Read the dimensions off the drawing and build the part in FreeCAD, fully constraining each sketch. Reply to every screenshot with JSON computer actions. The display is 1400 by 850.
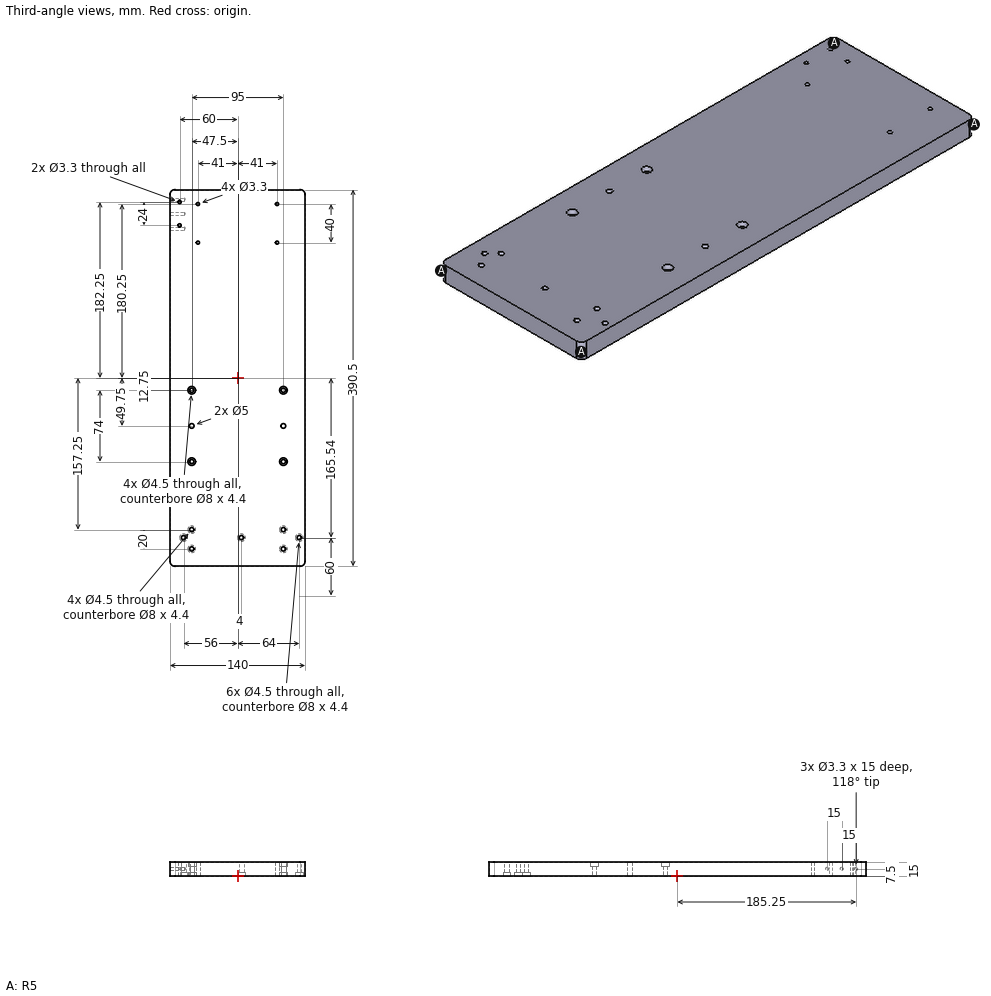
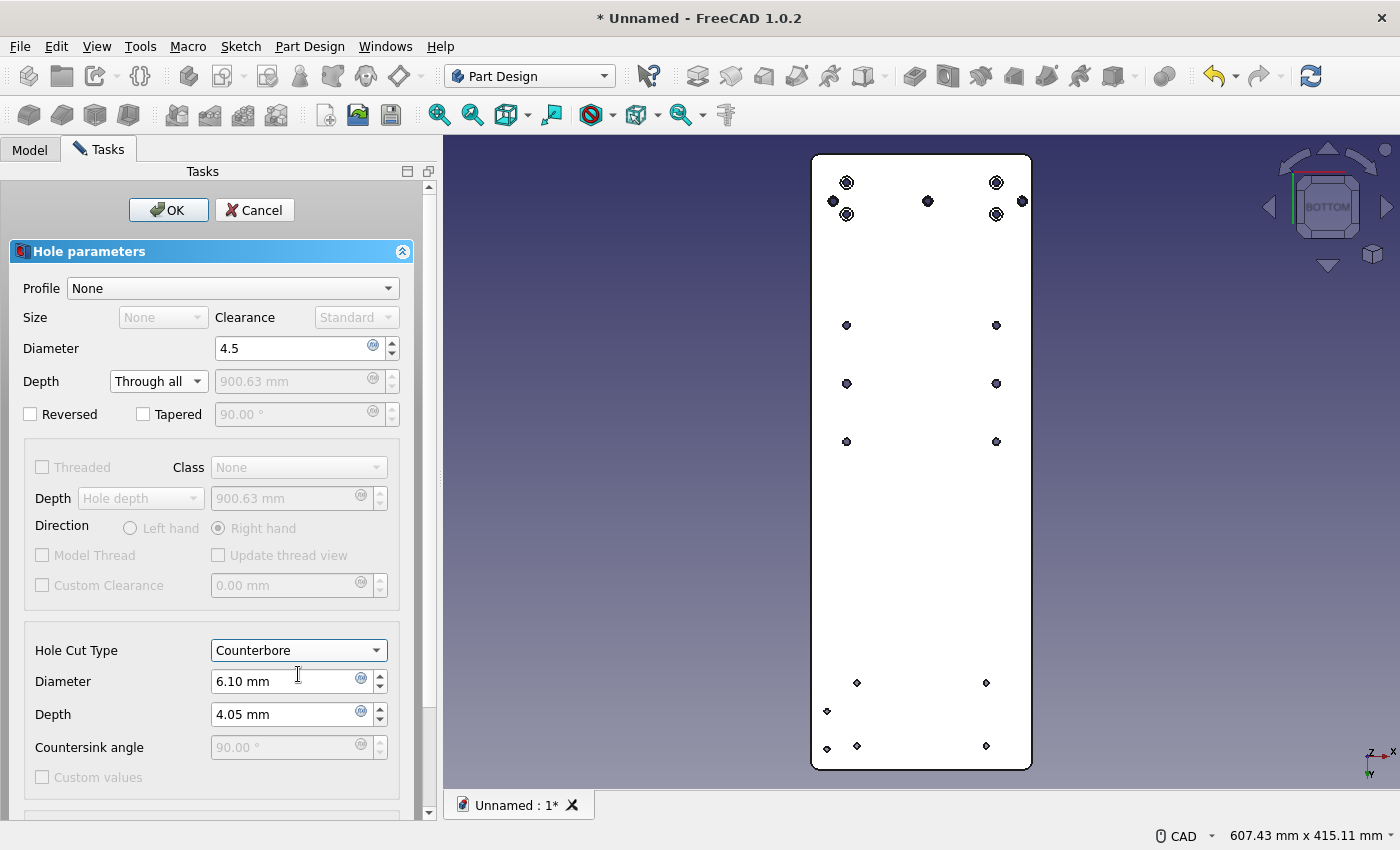
{"action": "triple_click", "coordinate": [292, 682]}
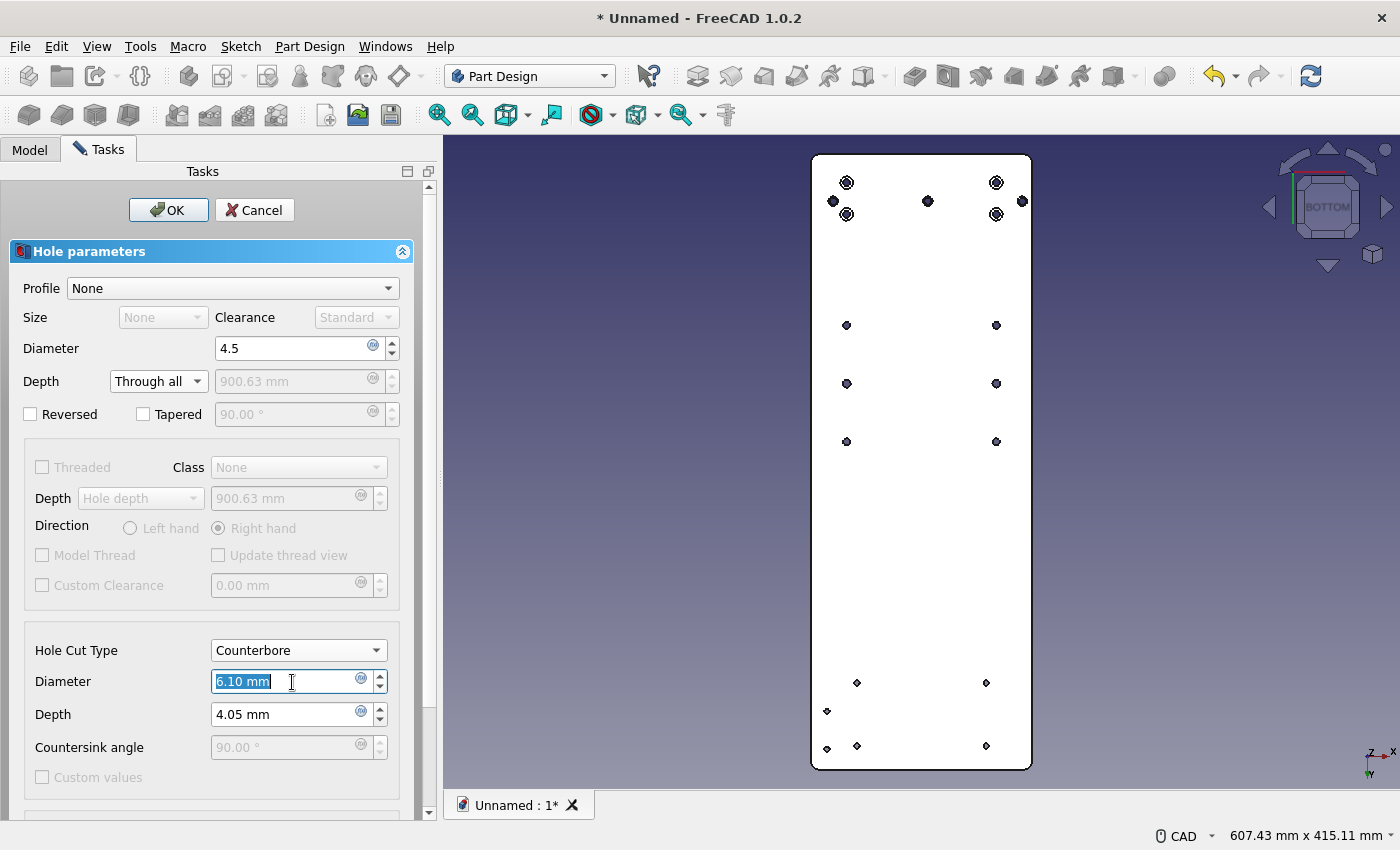
{"action": "type", "text": "8"}
{"action": "key", "text": "Tab"}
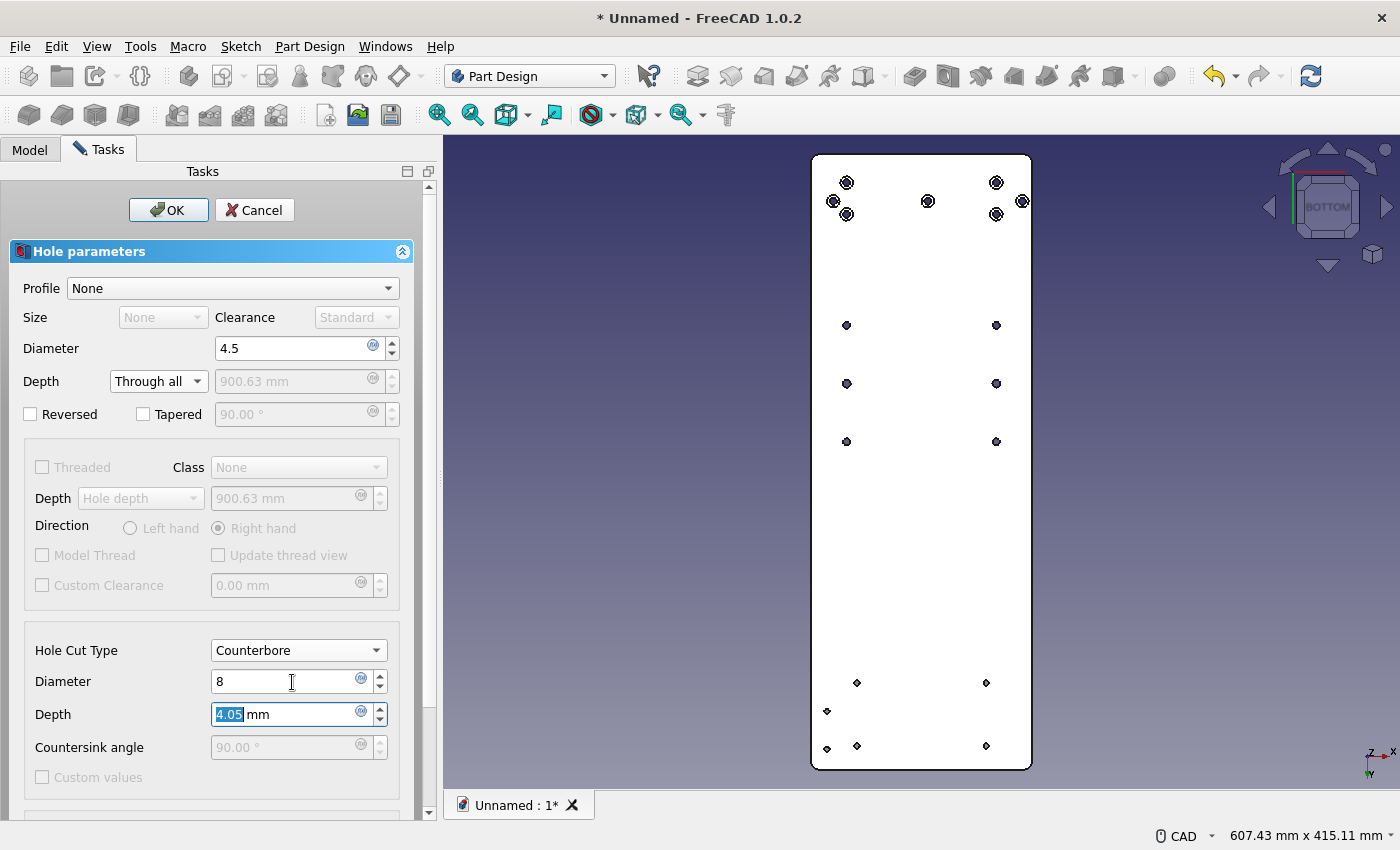
{"action": "type", "text": "4.4"}
{"action": "key", "text": "Tab"}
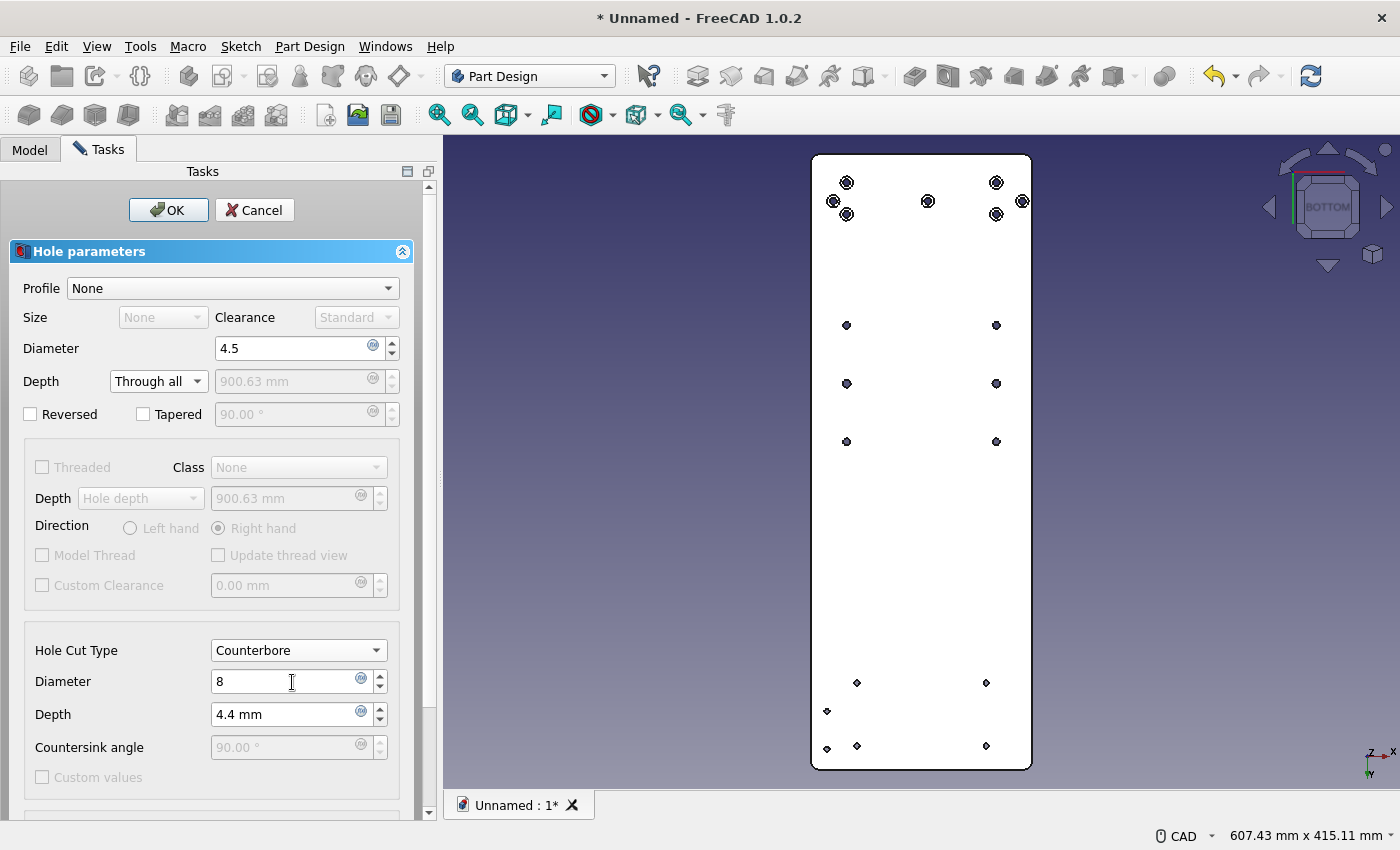
{"action": "left_click", "coordinate": [169, 210]}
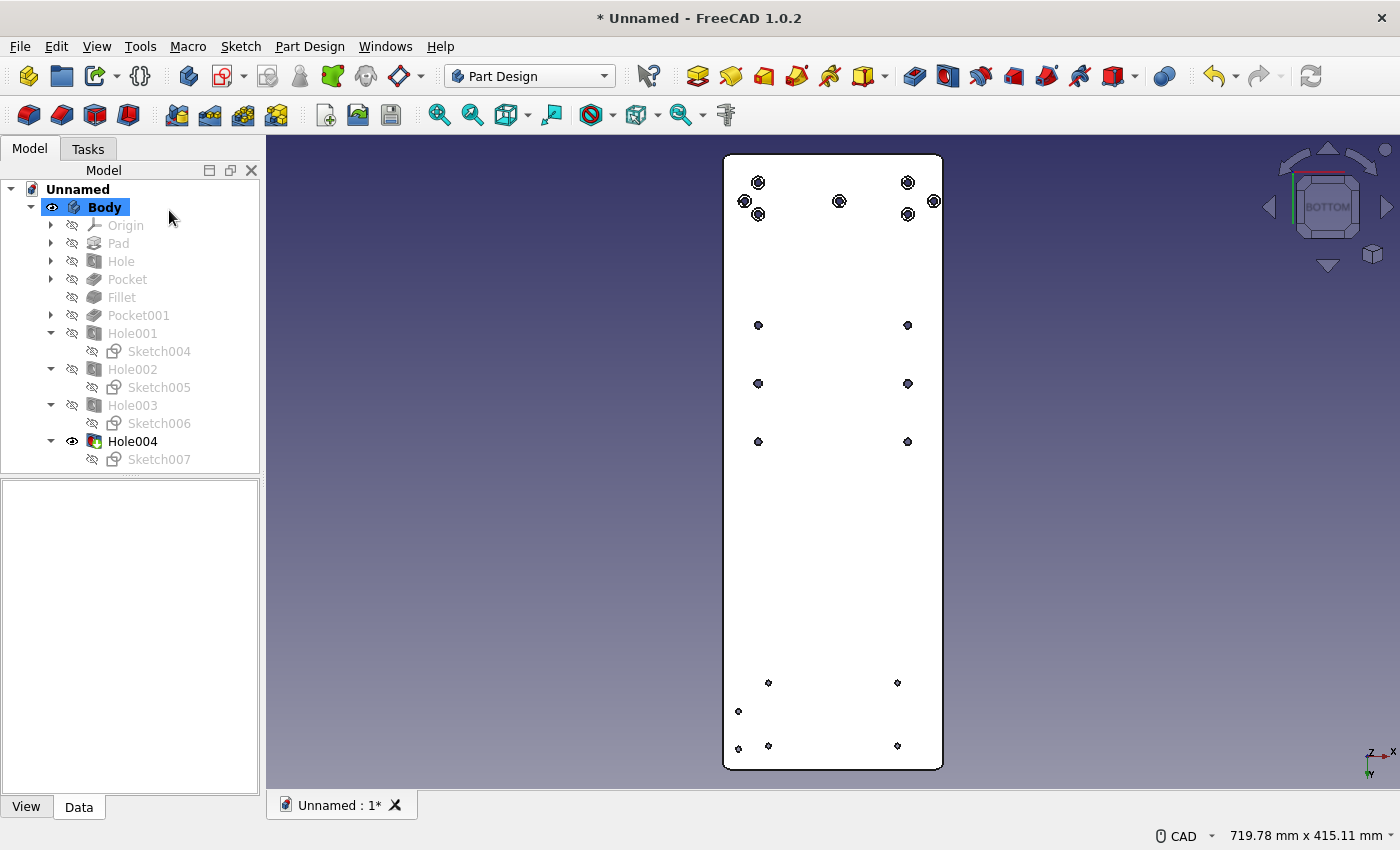
{"action": "key", "text": "0"}